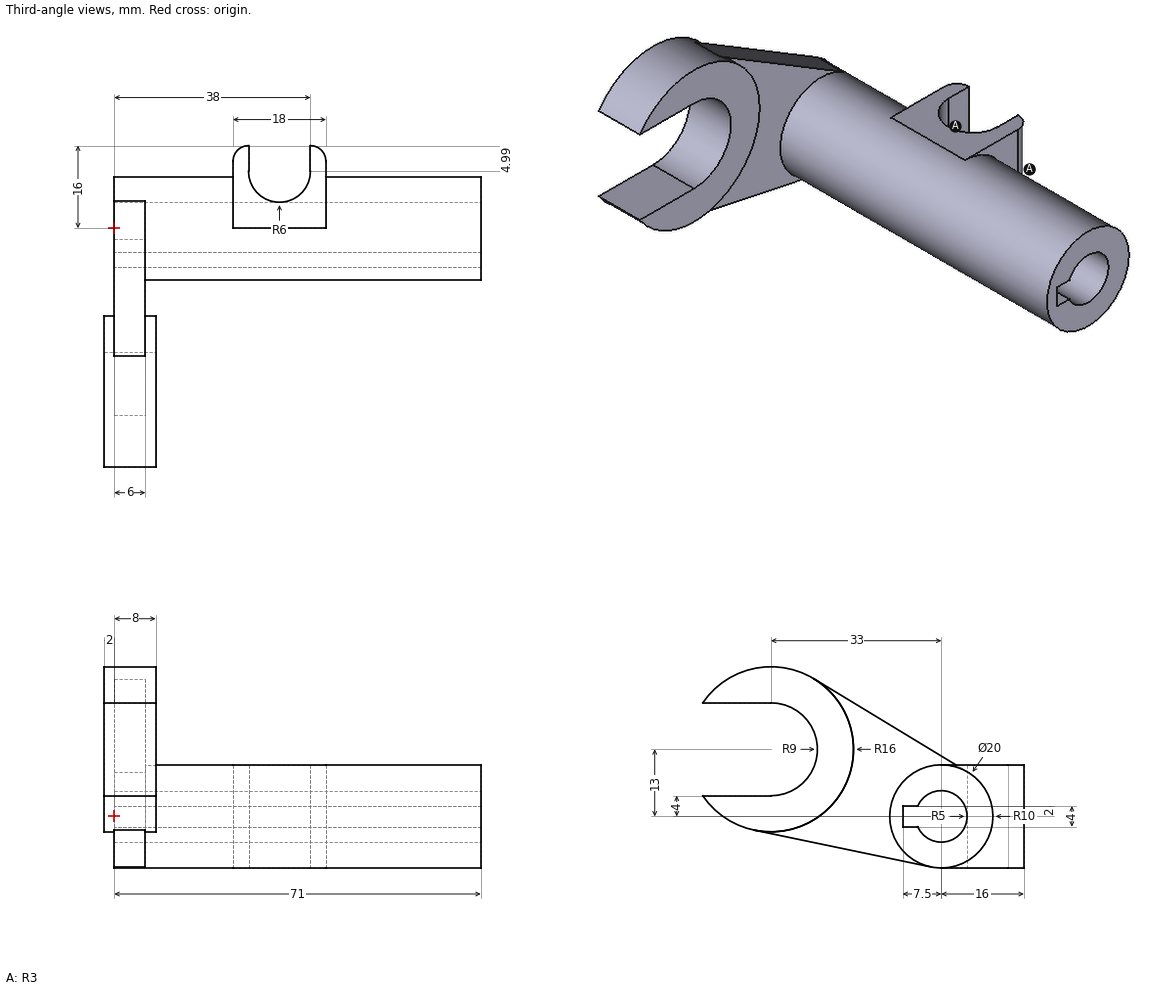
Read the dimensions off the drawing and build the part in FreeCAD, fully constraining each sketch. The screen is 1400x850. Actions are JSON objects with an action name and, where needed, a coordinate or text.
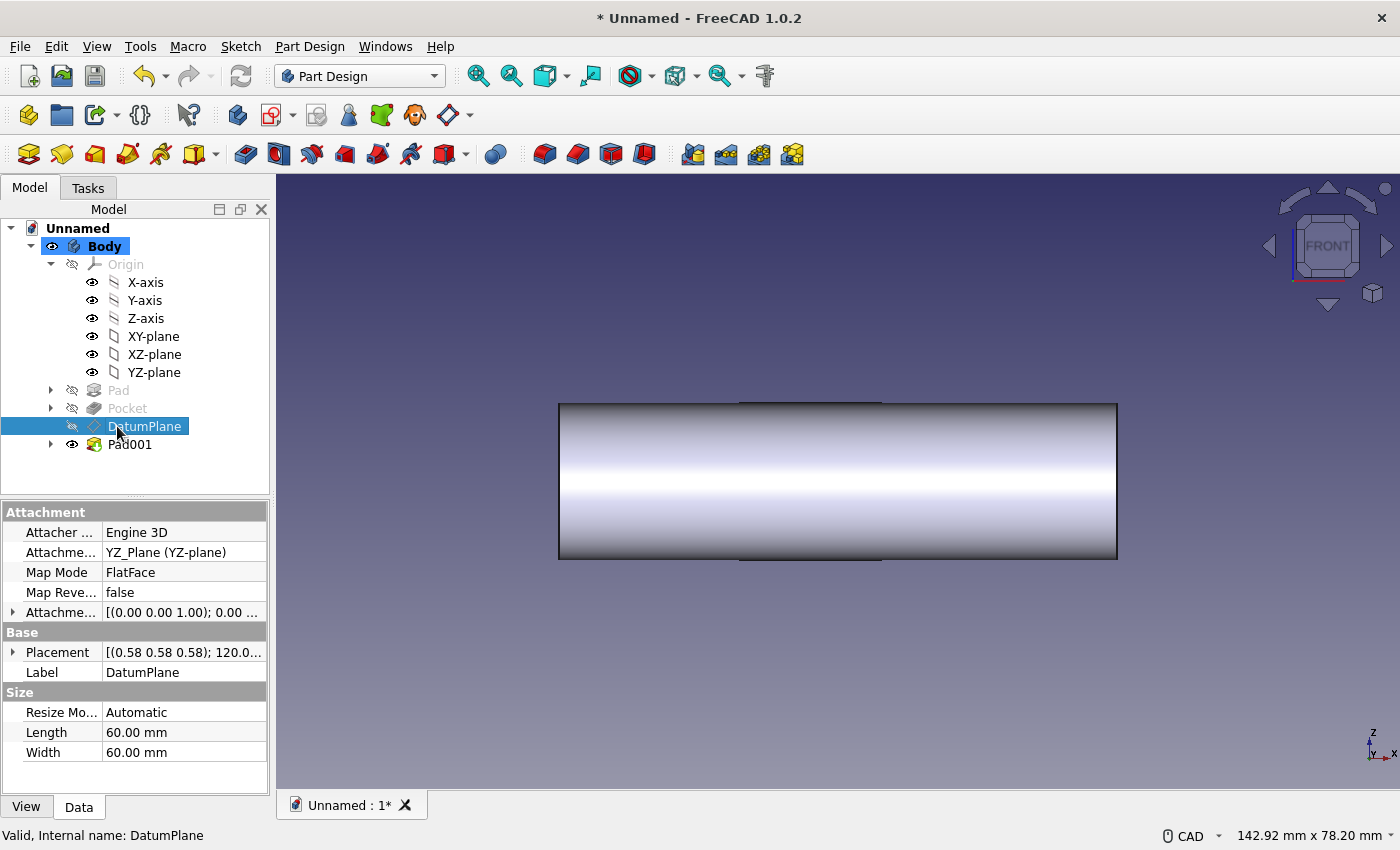
{"action": "key", "text": "3"}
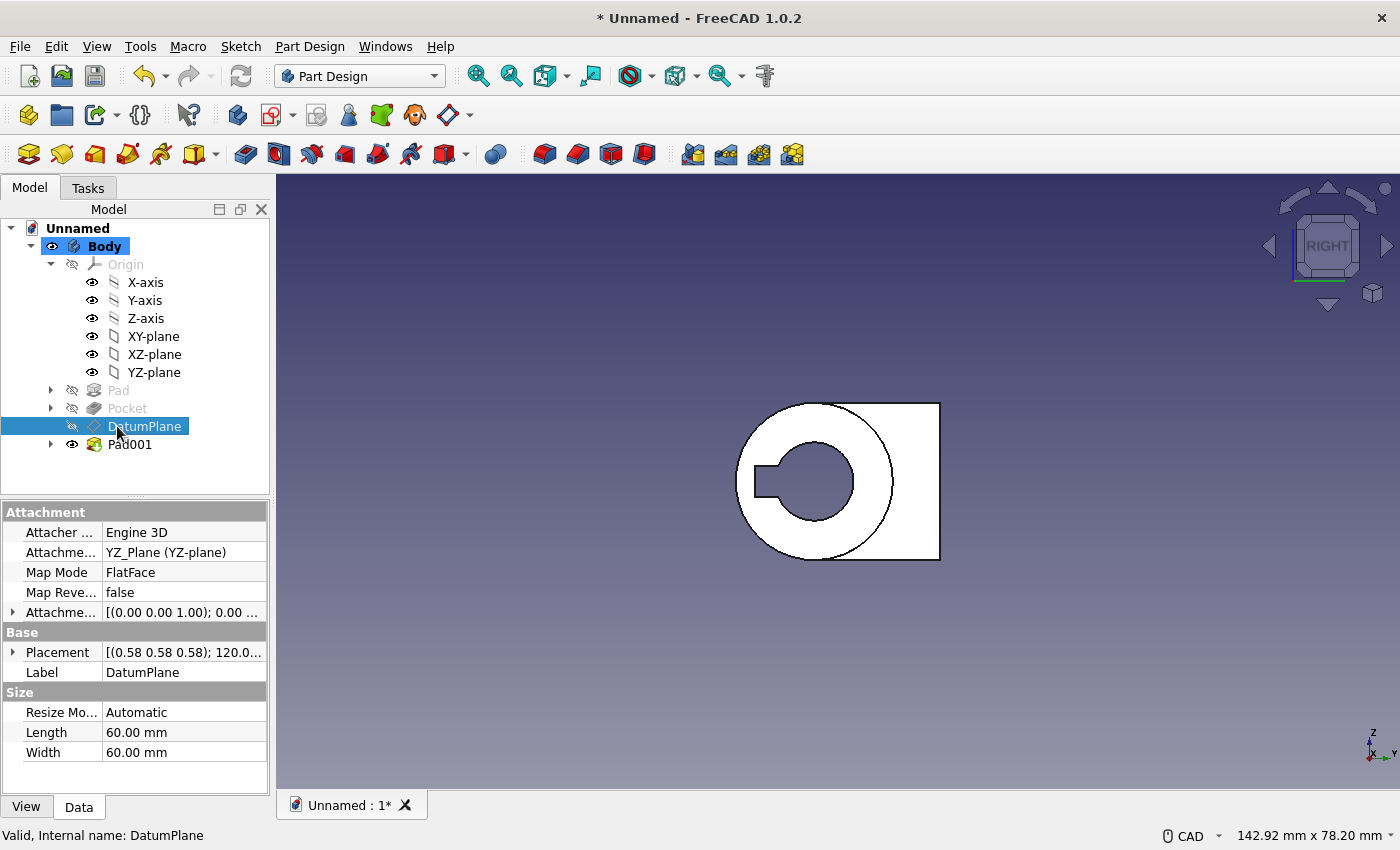
{"action": "key", "text": "v f"}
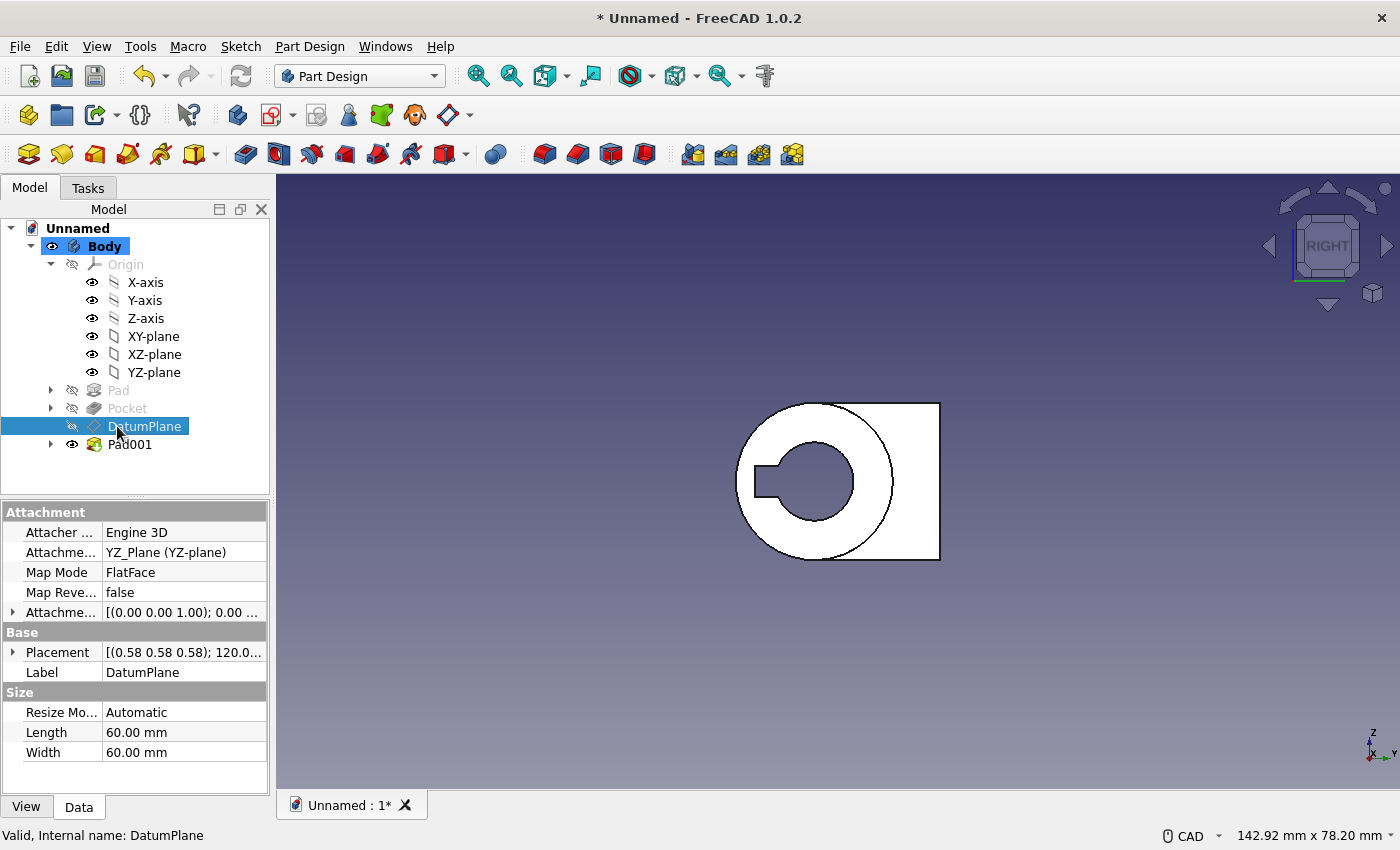
{"action": "left_click", "coordinate": [940, 480]}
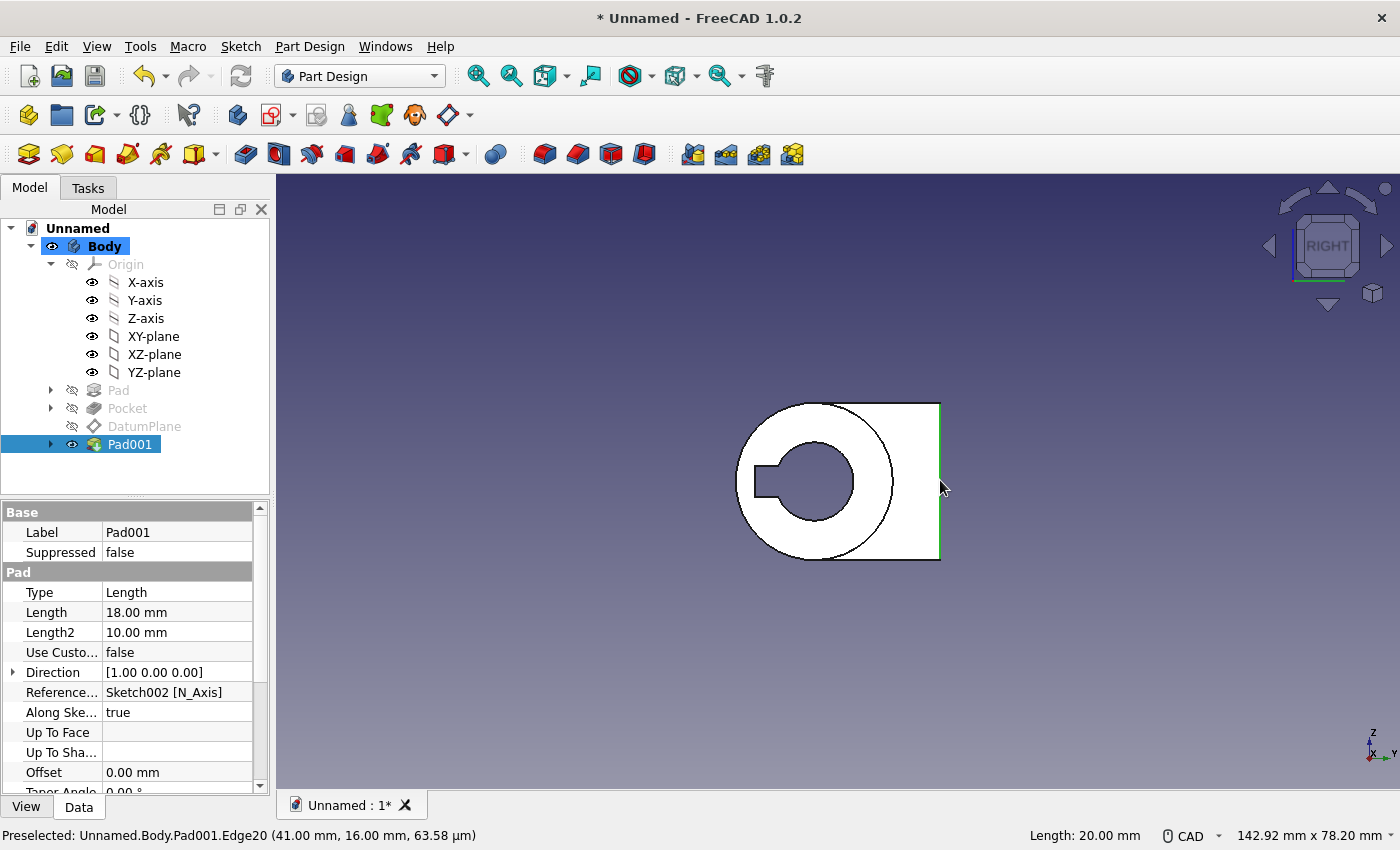
{"action": "key", "text": "5"}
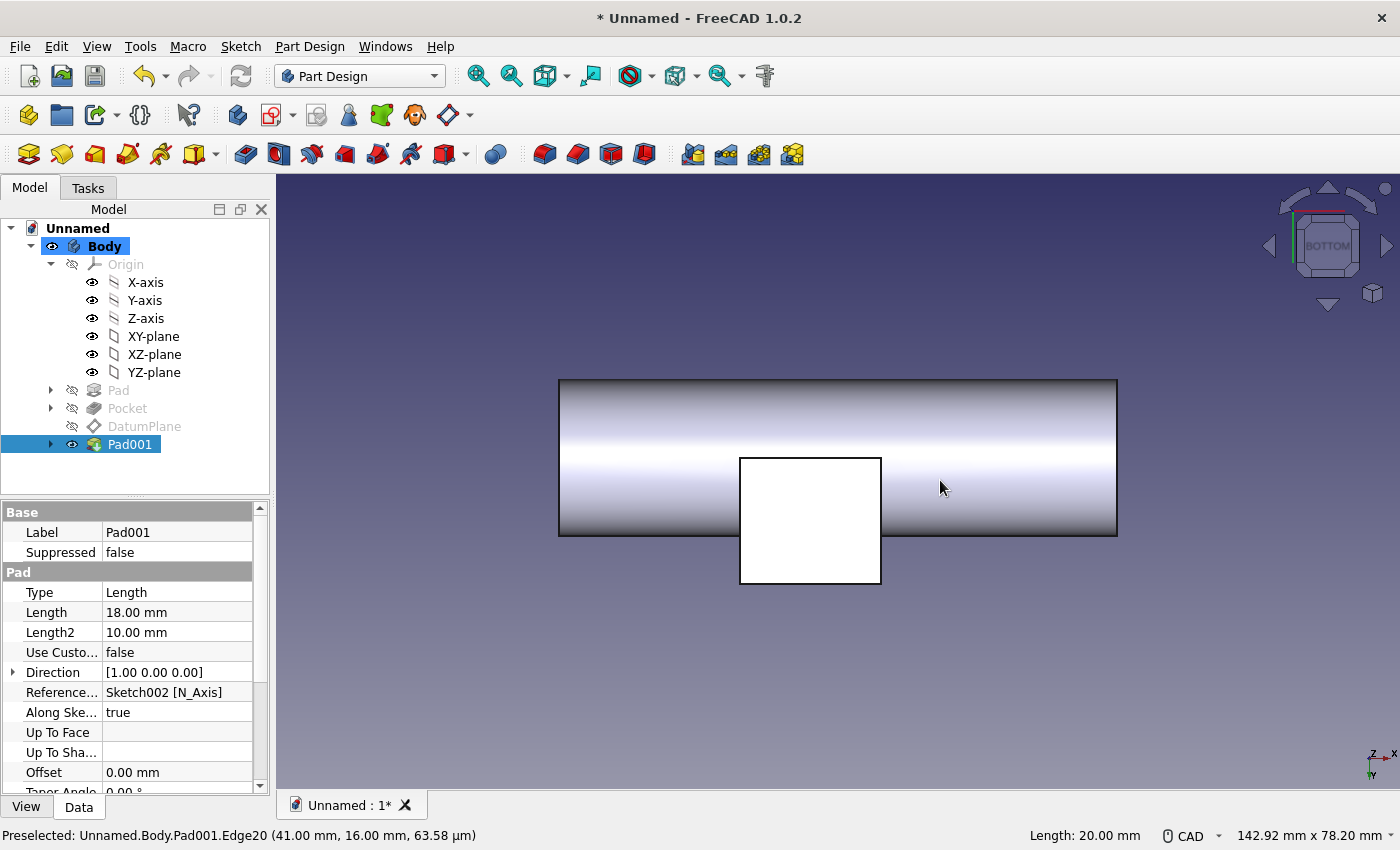
{"action": "key", "text": "4"}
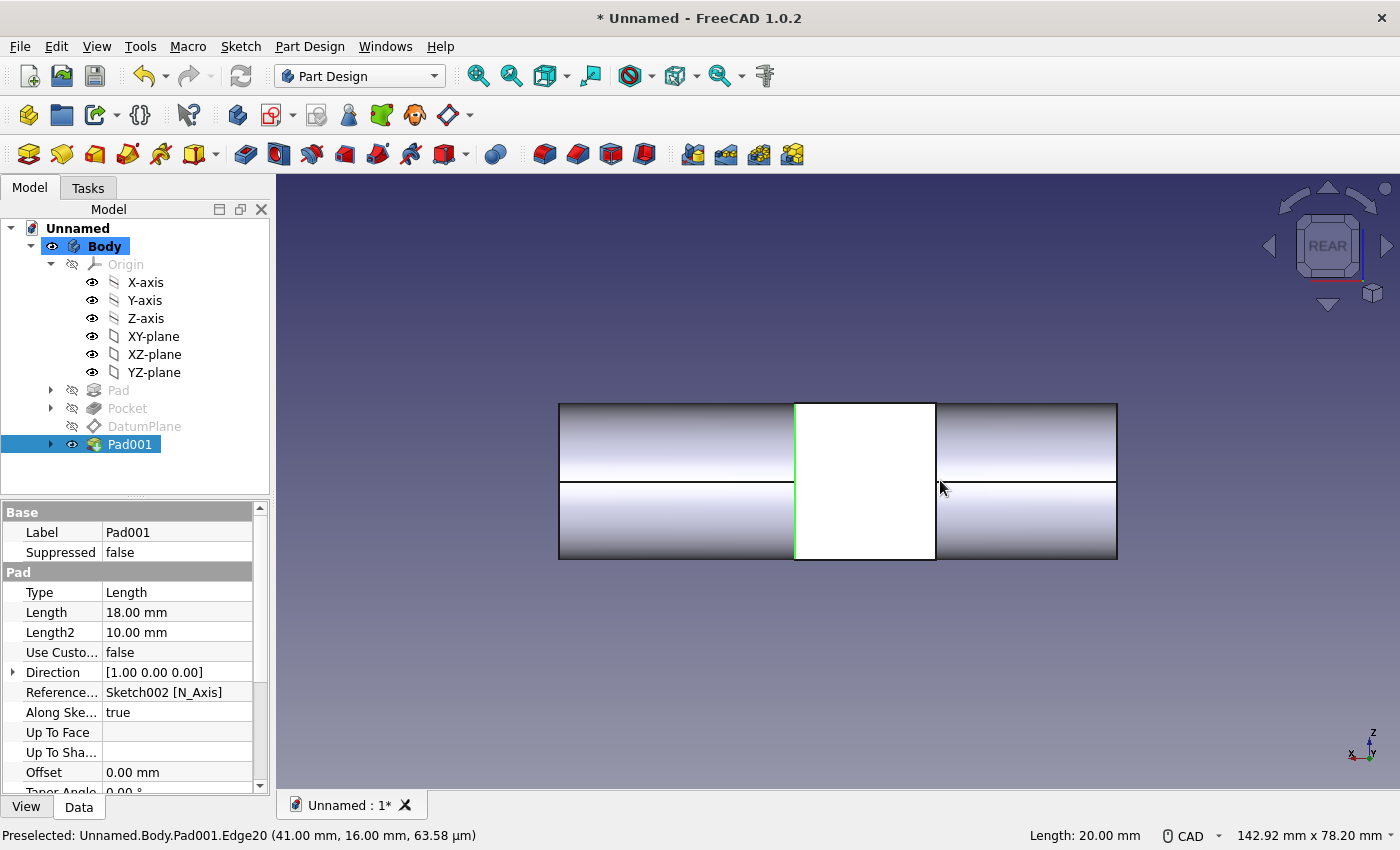
{"action": "left_click", "coordinate": [936, 481], "text": "ctrl"}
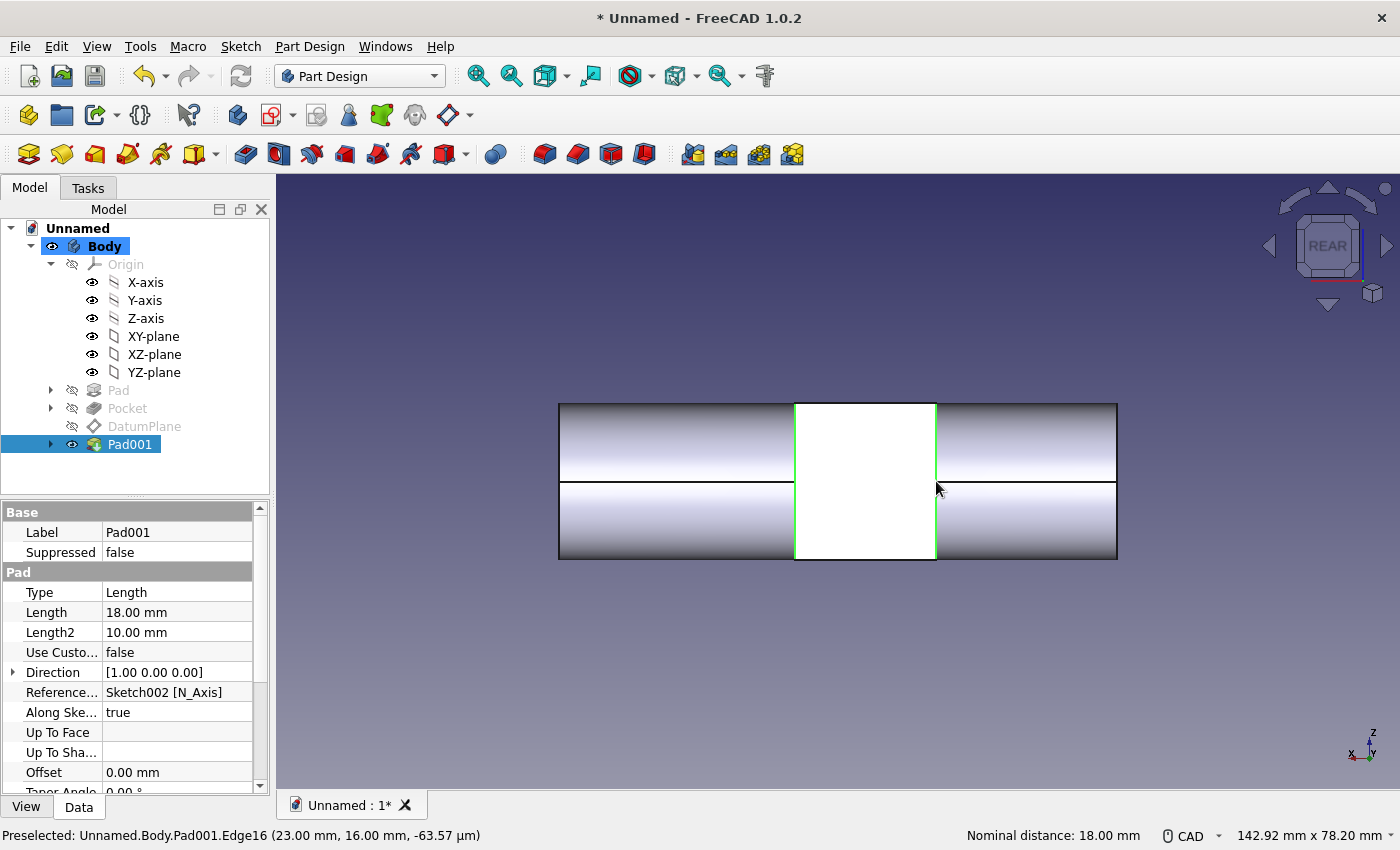
{"action": "left_click", "coordinate": [545, 154]}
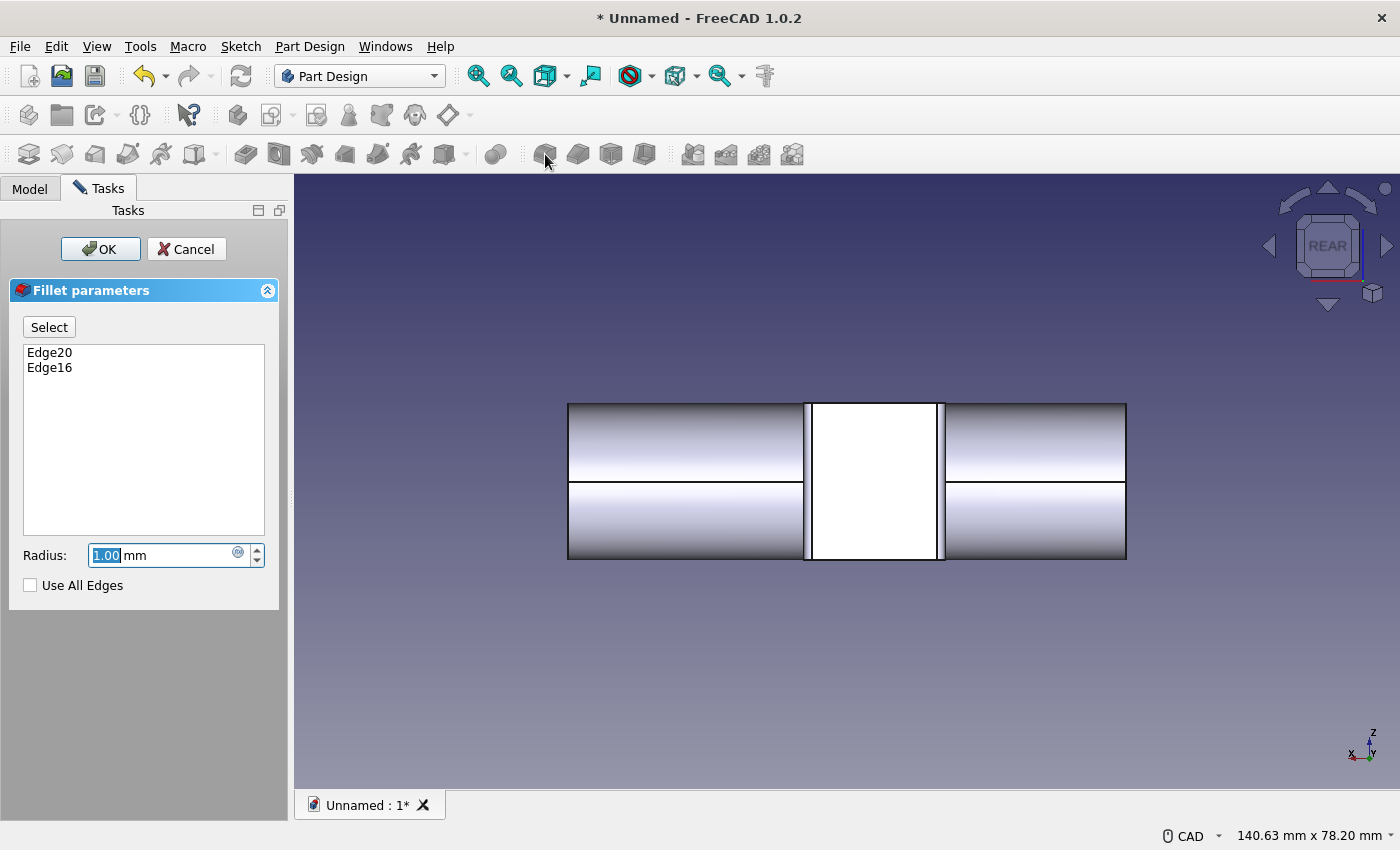
{"action": "type", "text": "3"}
{"action": "key", "text": "Tab"}